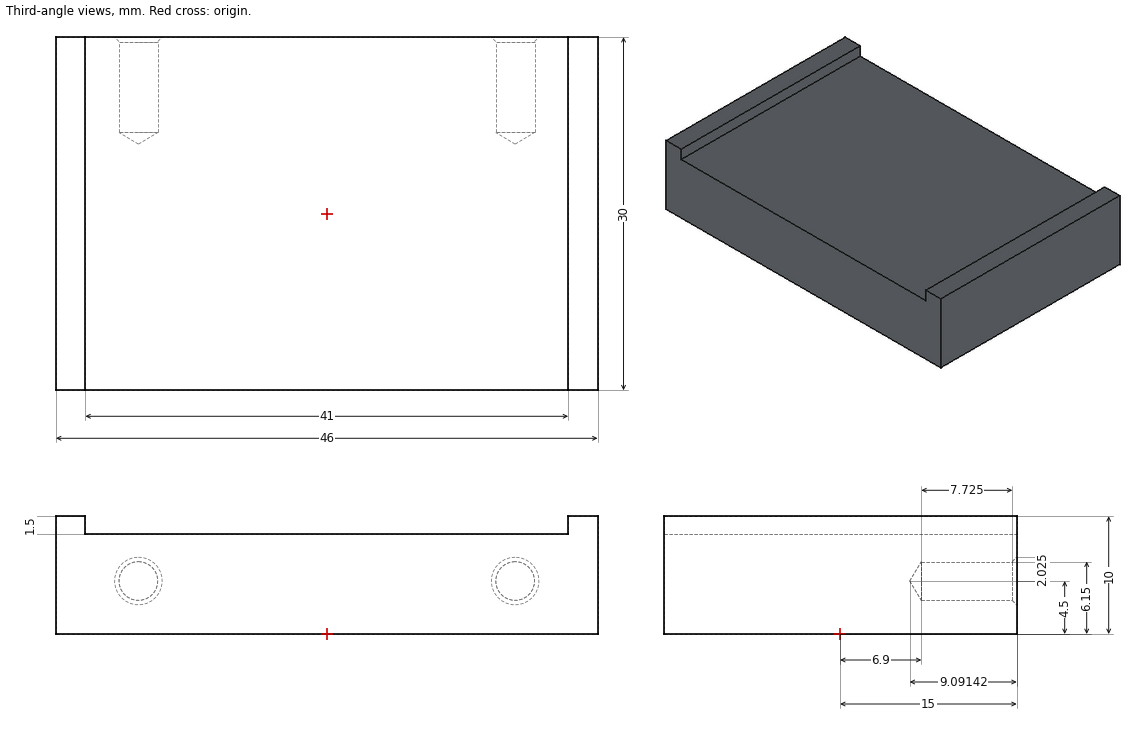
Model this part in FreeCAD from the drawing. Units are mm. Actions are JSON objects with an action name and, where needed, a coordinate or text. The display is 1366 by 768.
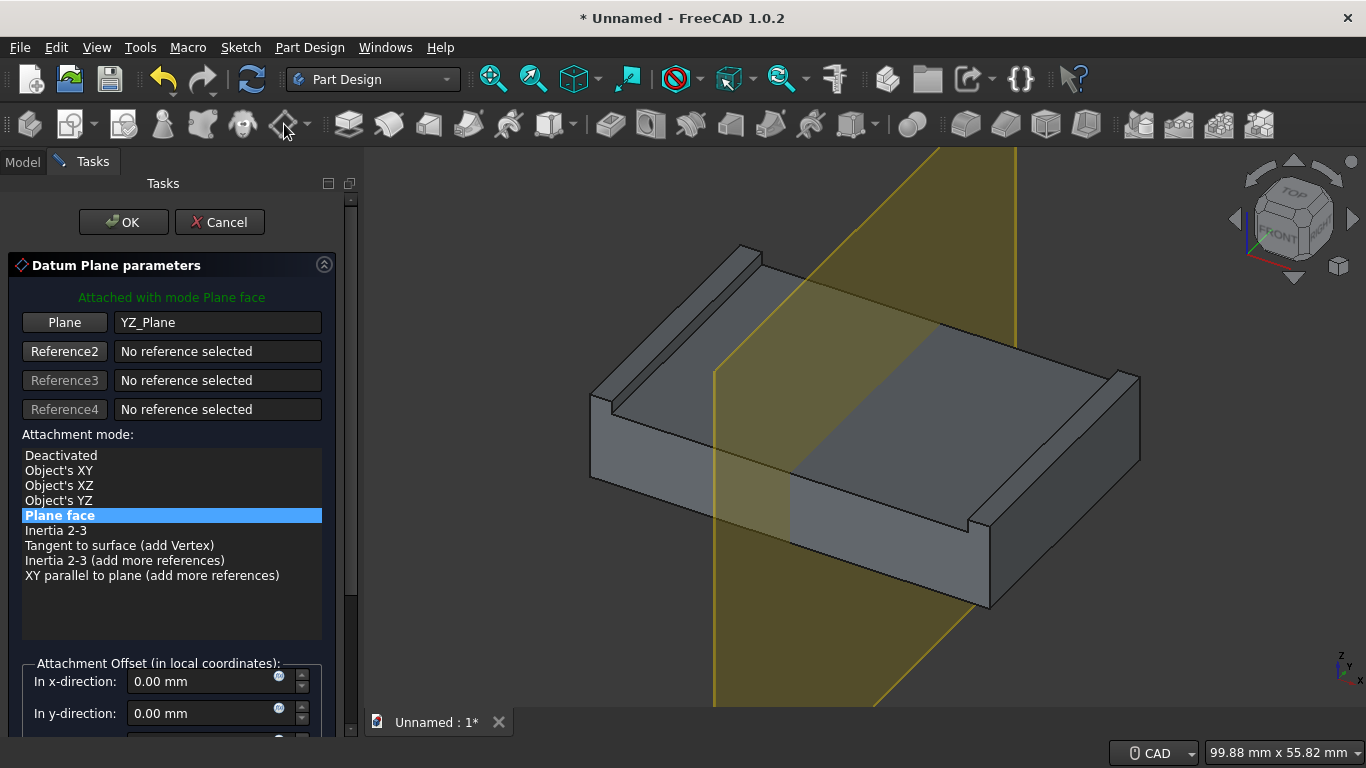
{"action": "scroll", "coordinate": [351, 464], "scroll_direction": "down", "scroll_amount": 2}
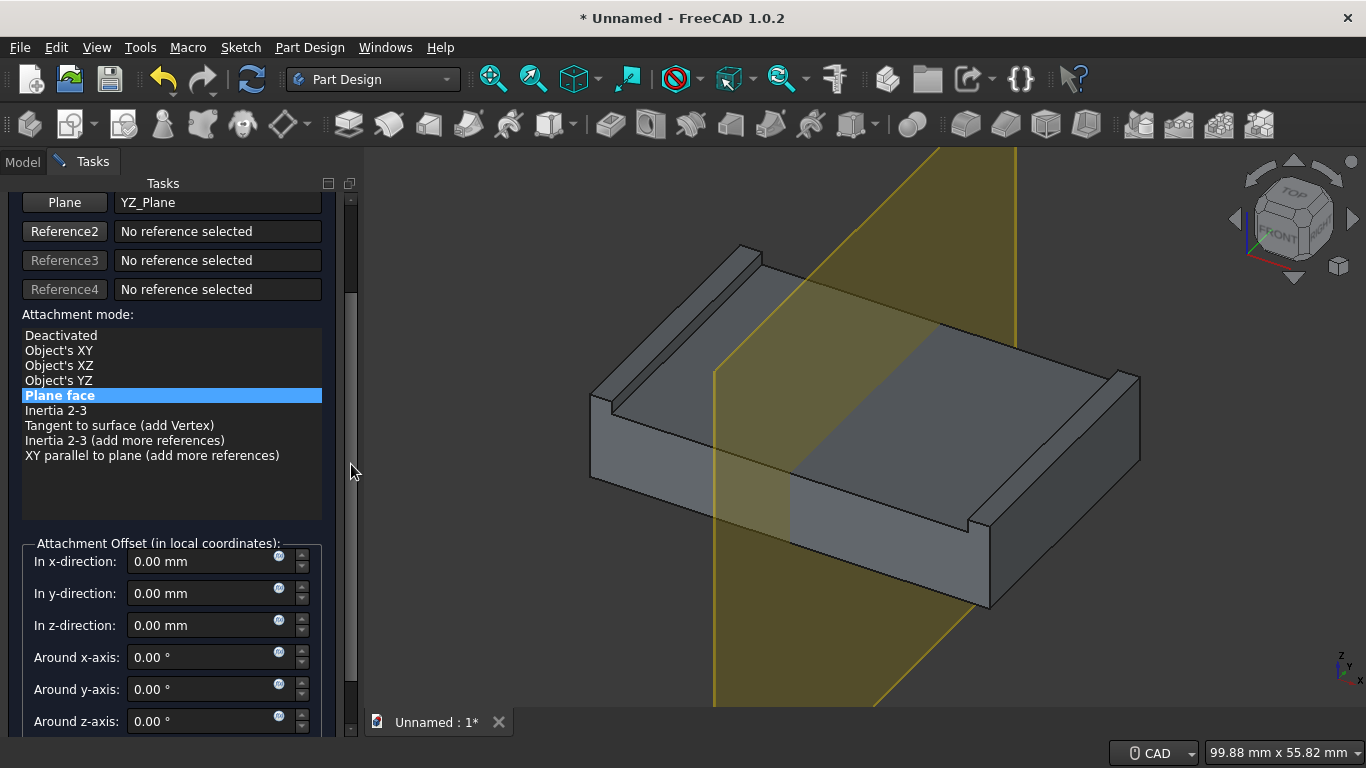
{"action": "triple_click", "coordinate": [210, 625]}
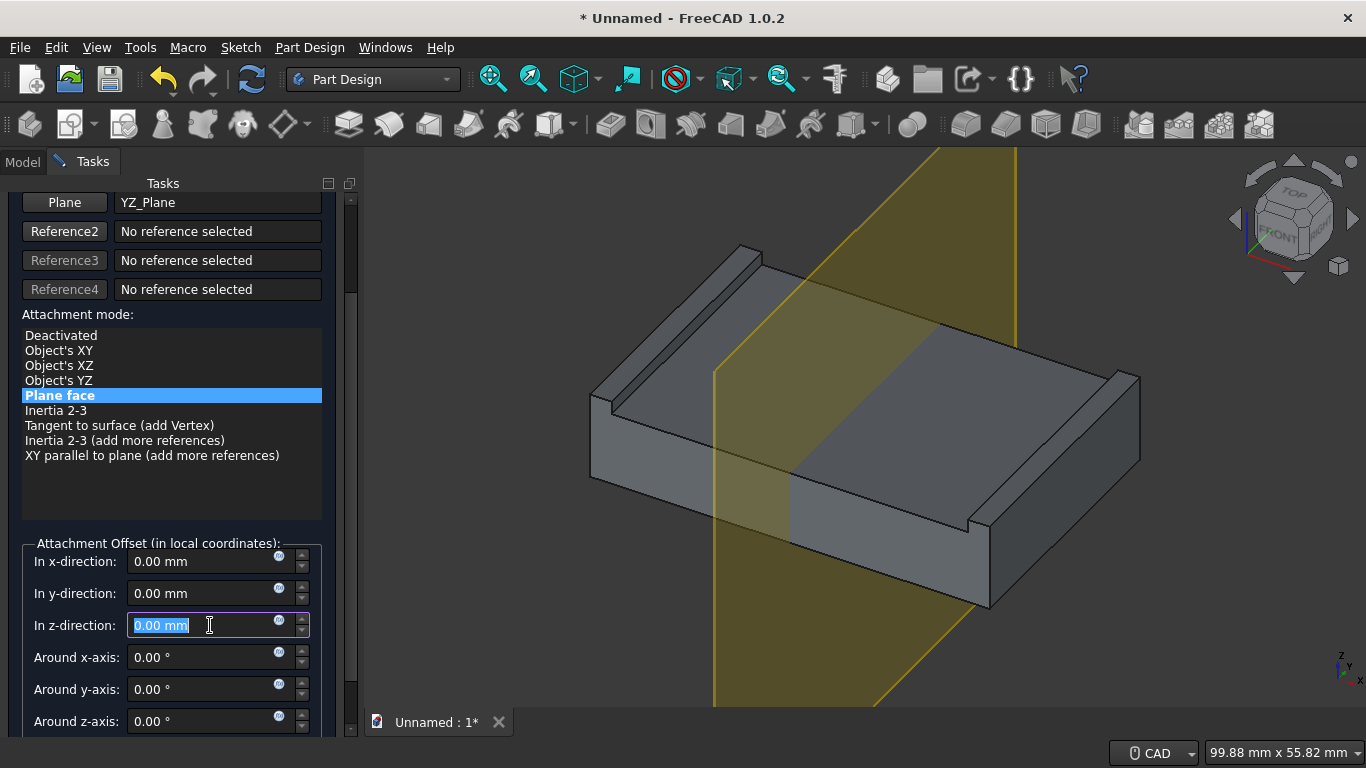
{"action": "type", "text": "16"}
{"action": "key", "text": "Tab"}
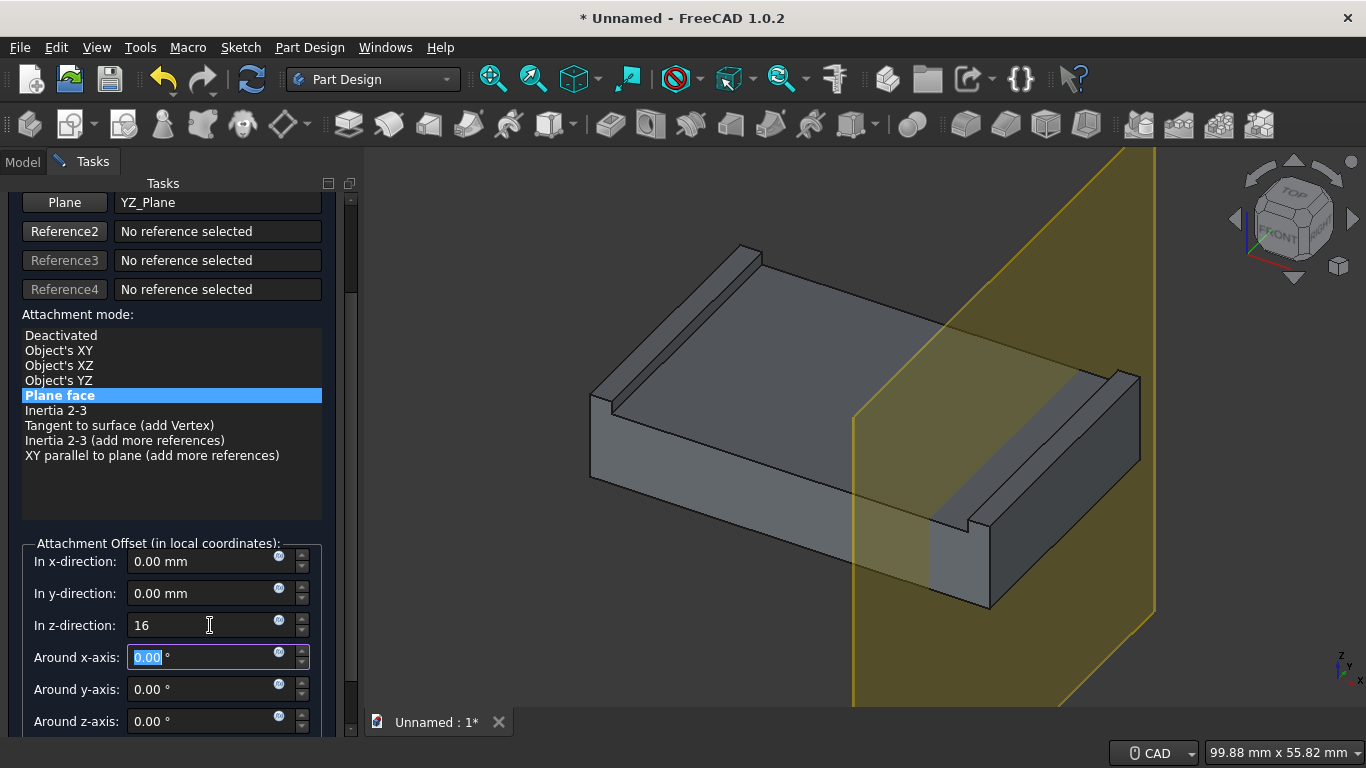
{"action": "scroll", "coordinate": [351, 464], "scroll_direction": "up", "scroll_amount": 3}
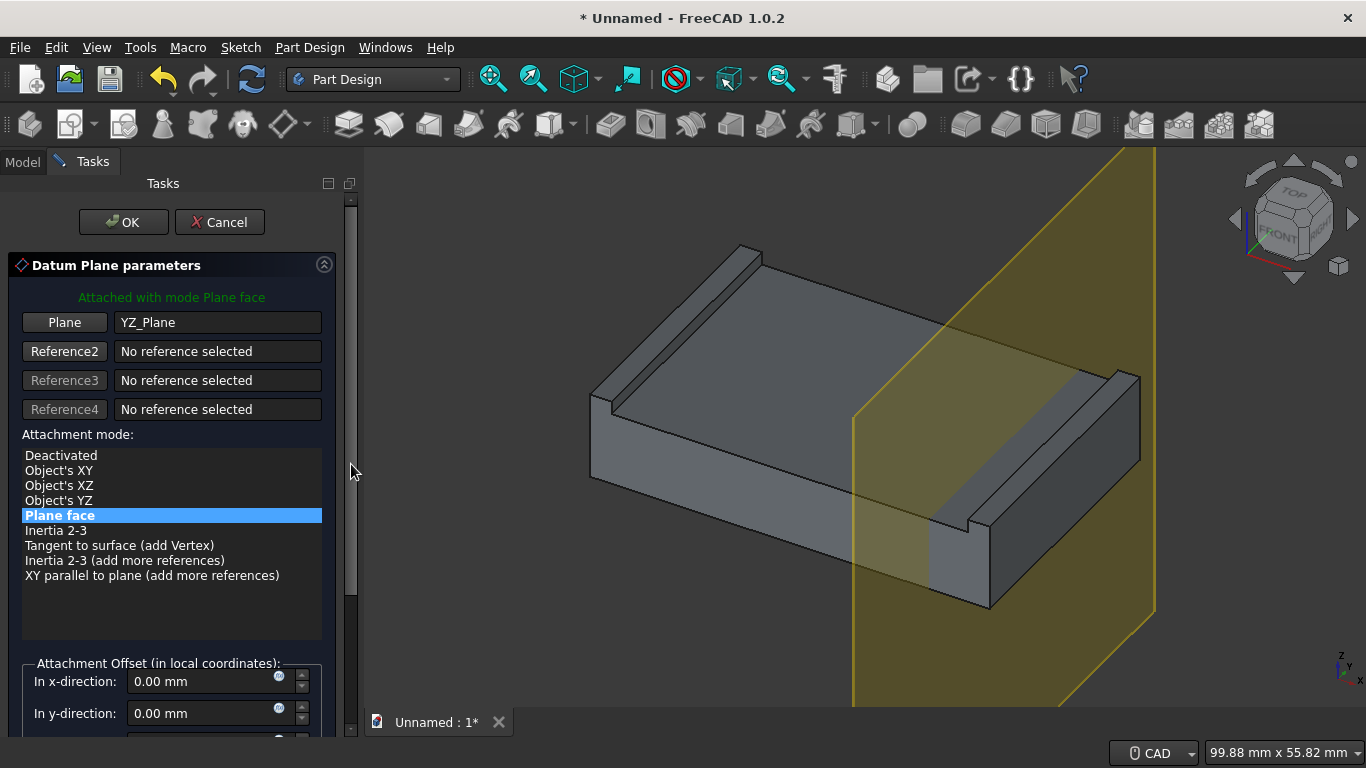
{"action": "left_click", "coordinate": [124, 222]}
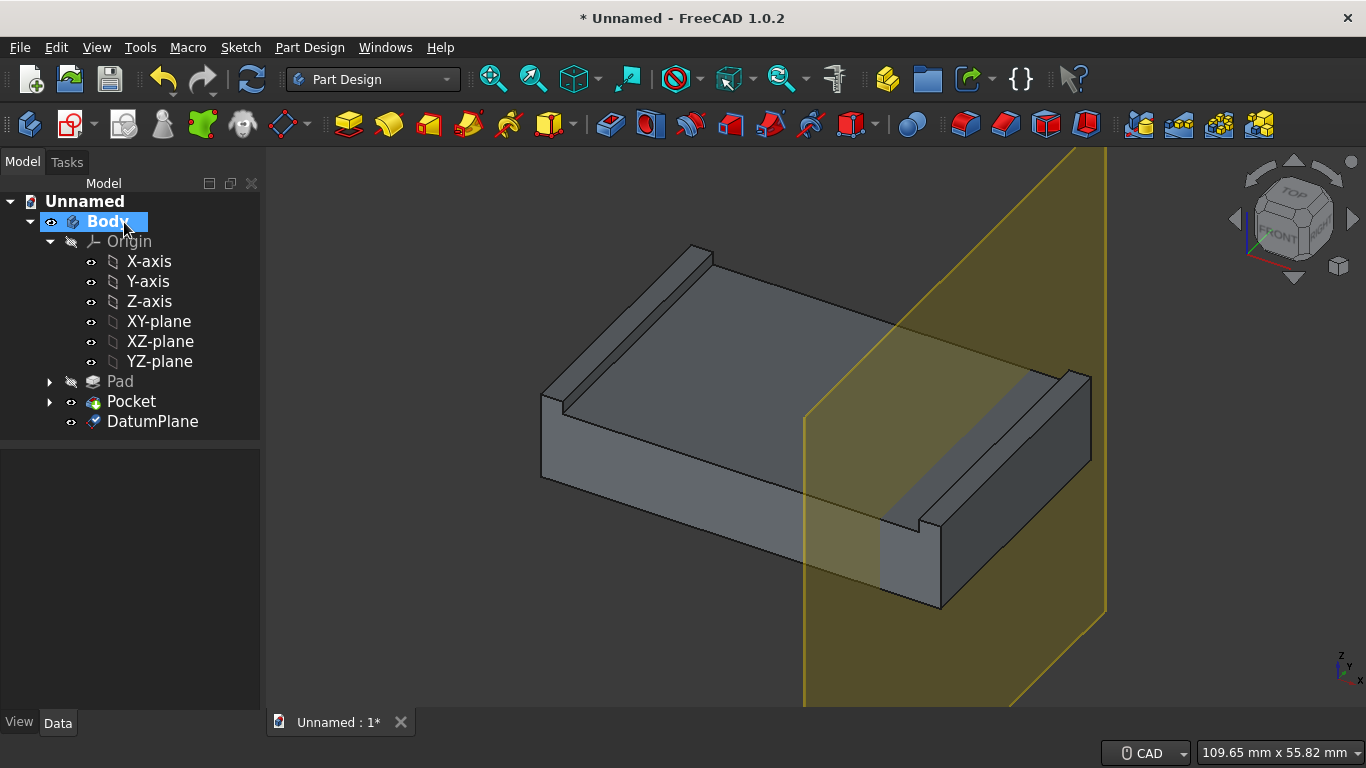
{"action": "left_click", "coordinate": [116, 422]}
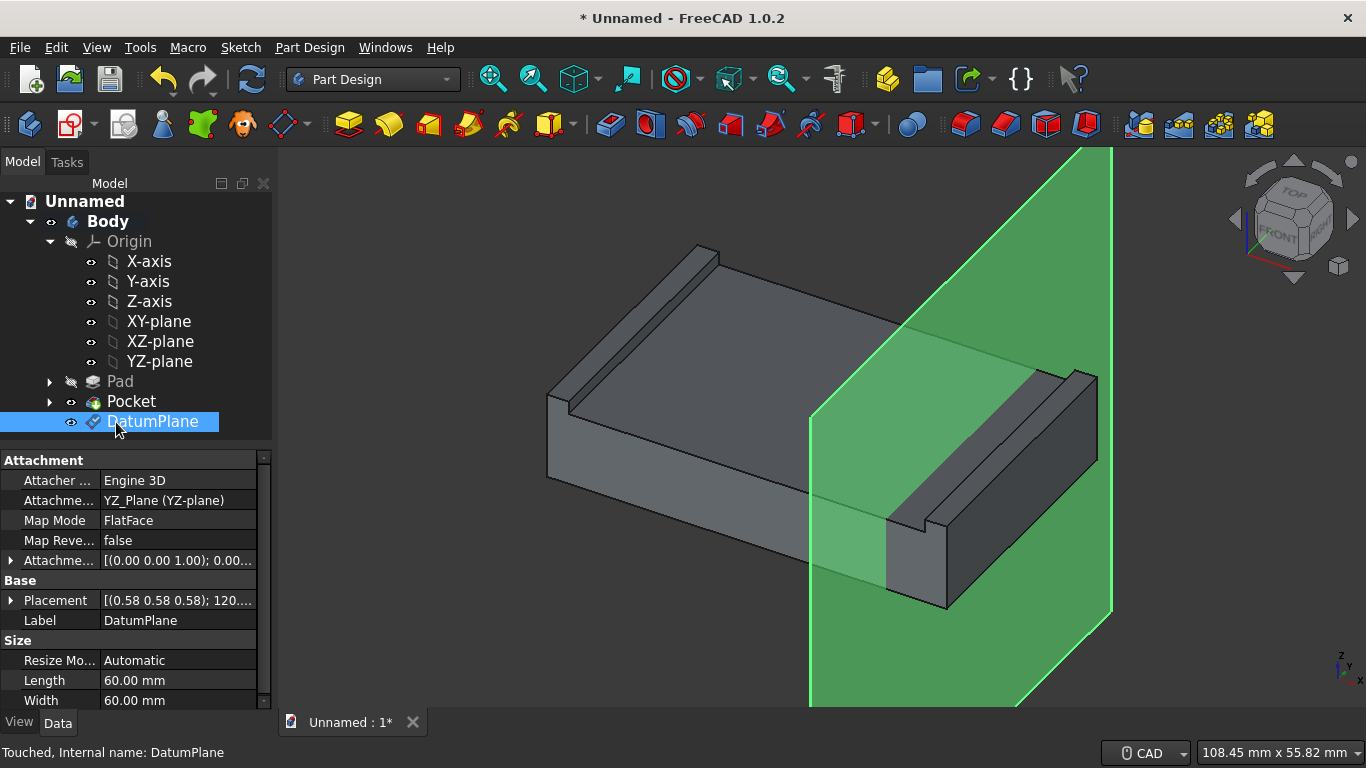
{"action": "left_click", "coordinate": [70, 124]}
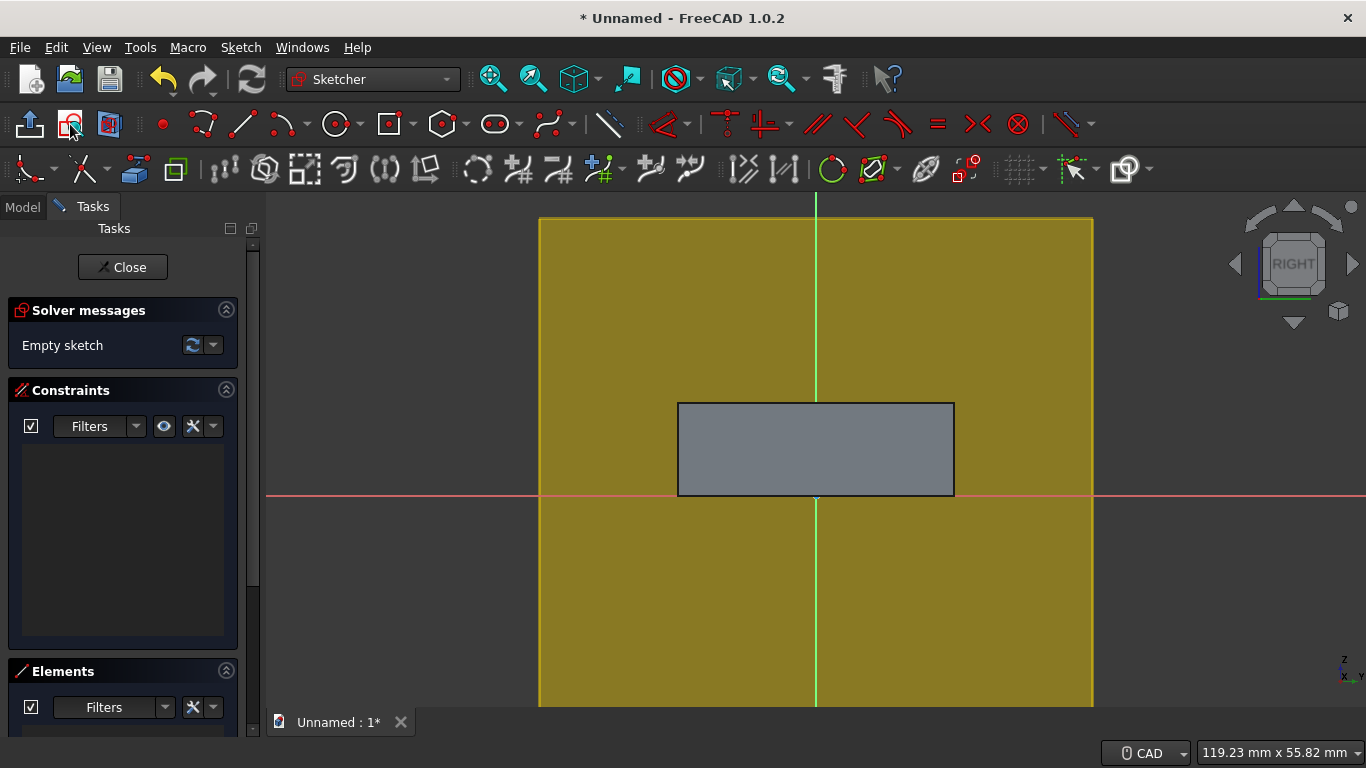
{"action": "key", "text": "q s"}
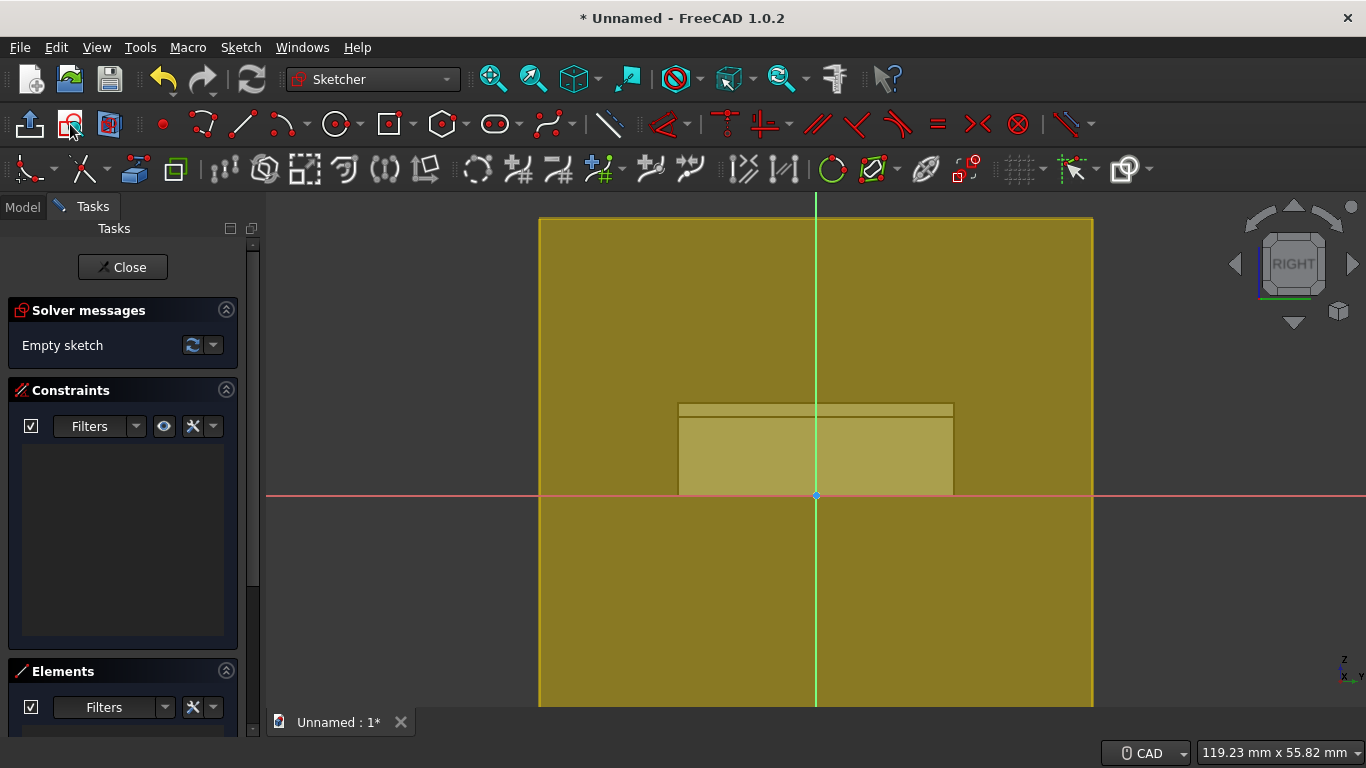
{"action": "scroll", "coordinate": [920, 470], "scroll_direction": "up", "scroll_amount": 8}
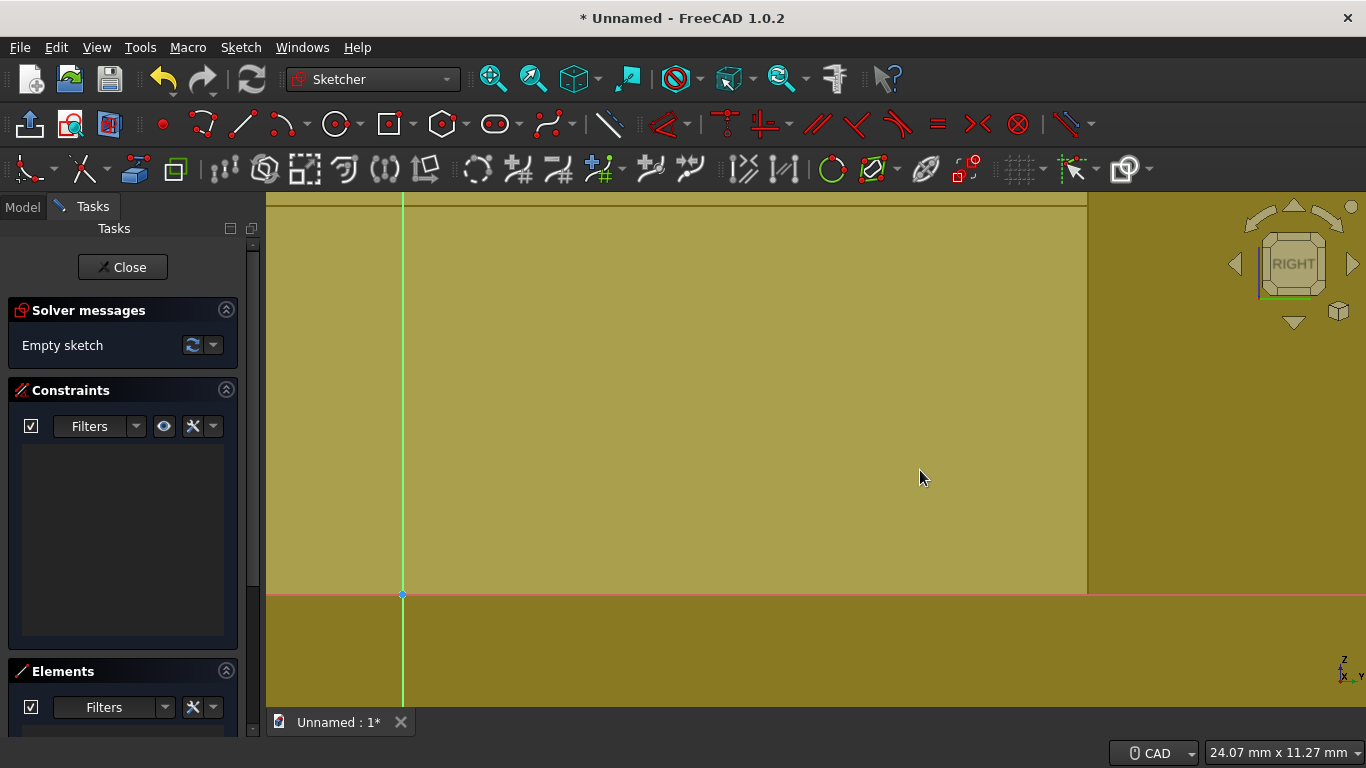
{"action": "left_click", "coordinate": [204, 124]}